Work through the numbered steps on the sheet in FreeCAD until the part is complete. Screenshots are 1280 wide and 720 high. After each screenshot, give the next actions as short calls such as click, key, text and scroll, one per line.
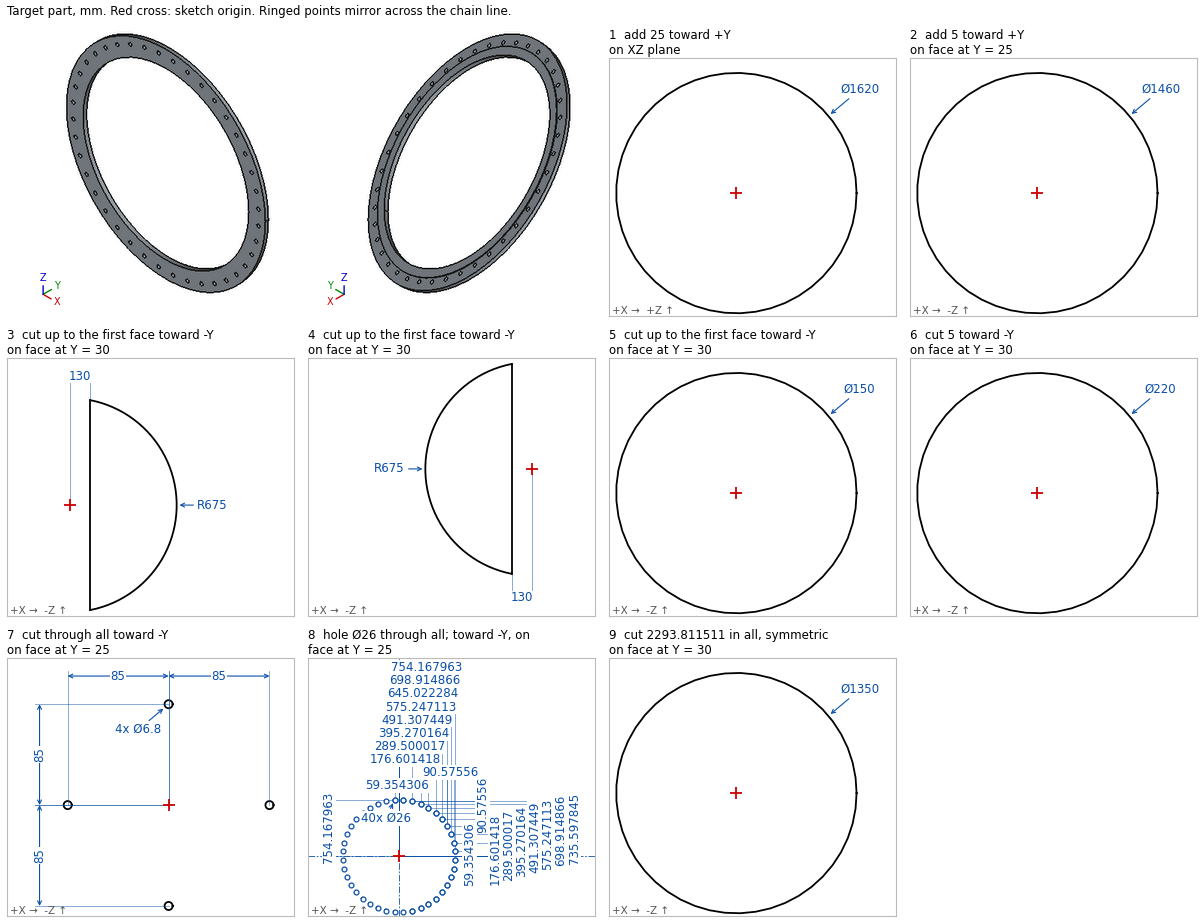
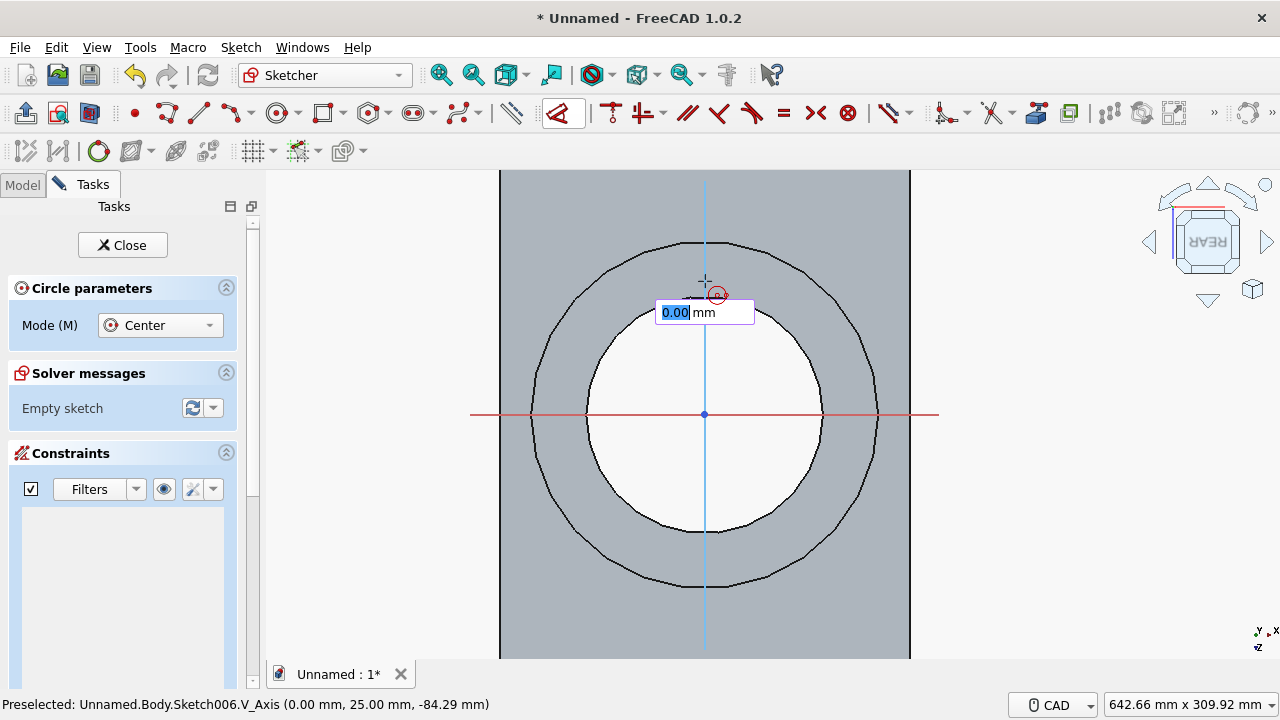
scroll(710, 279, up, 6)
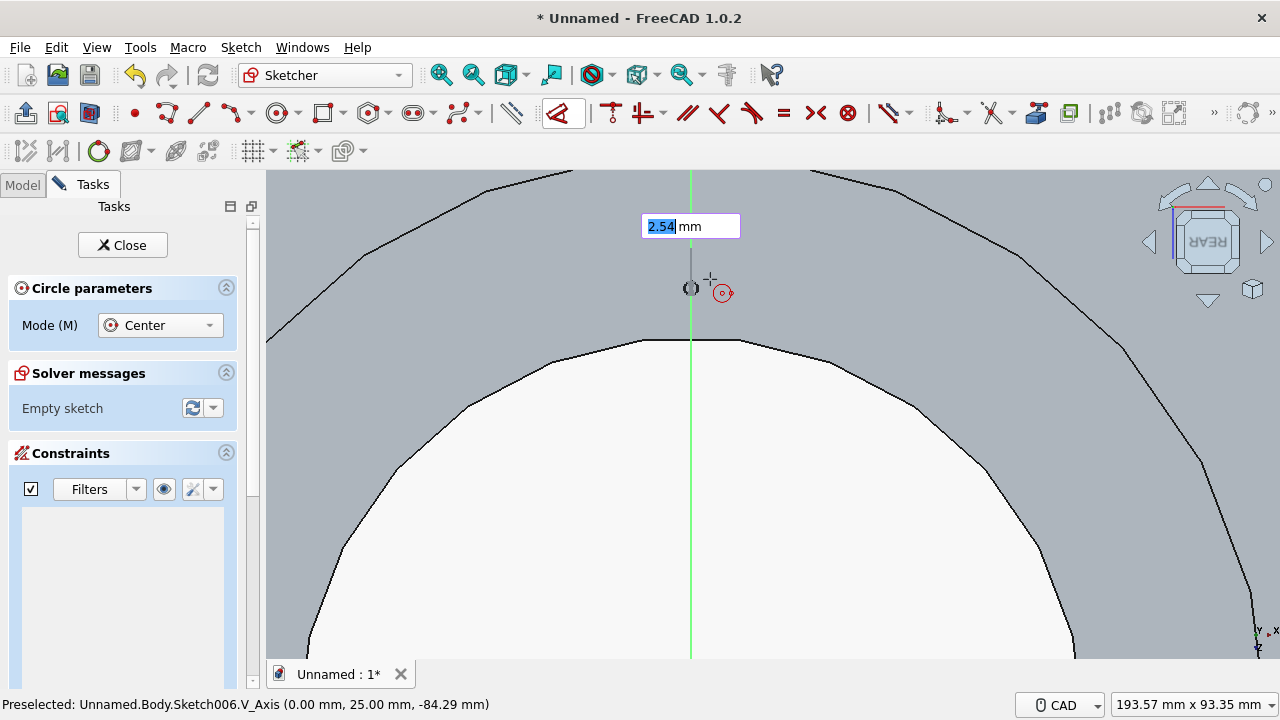
click(708, 279)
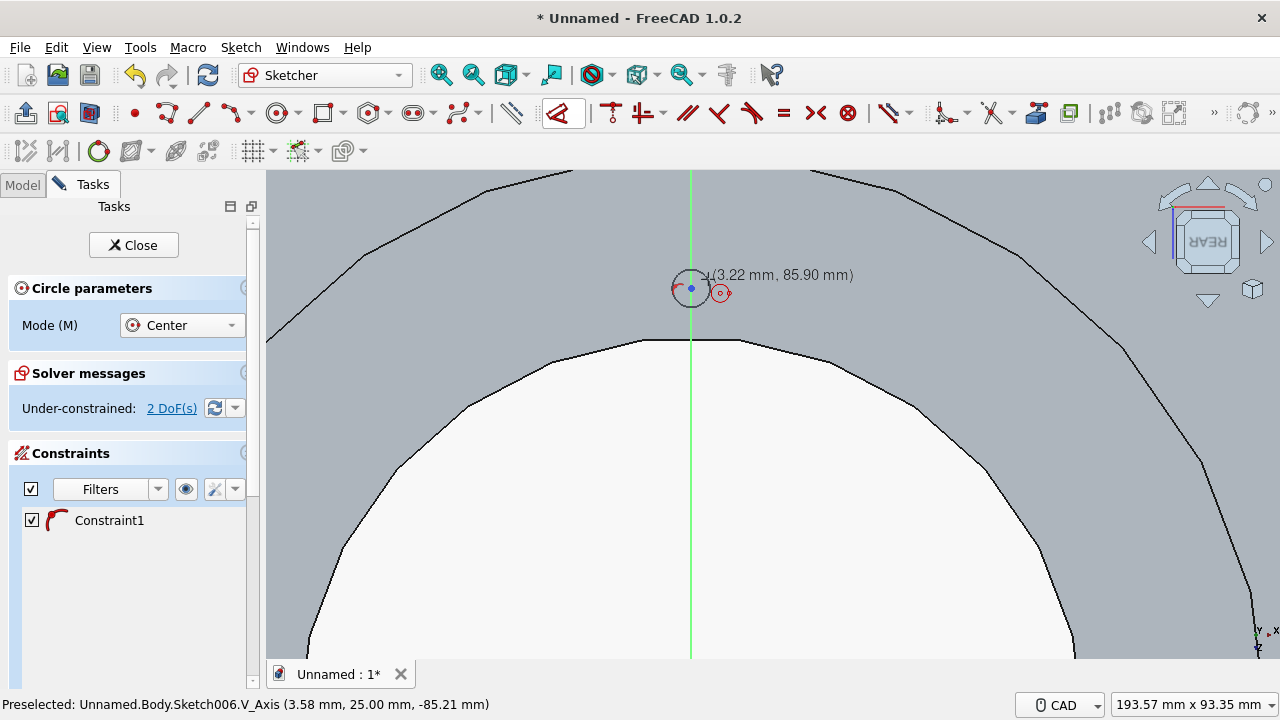
scroll(710, 279, down, 6)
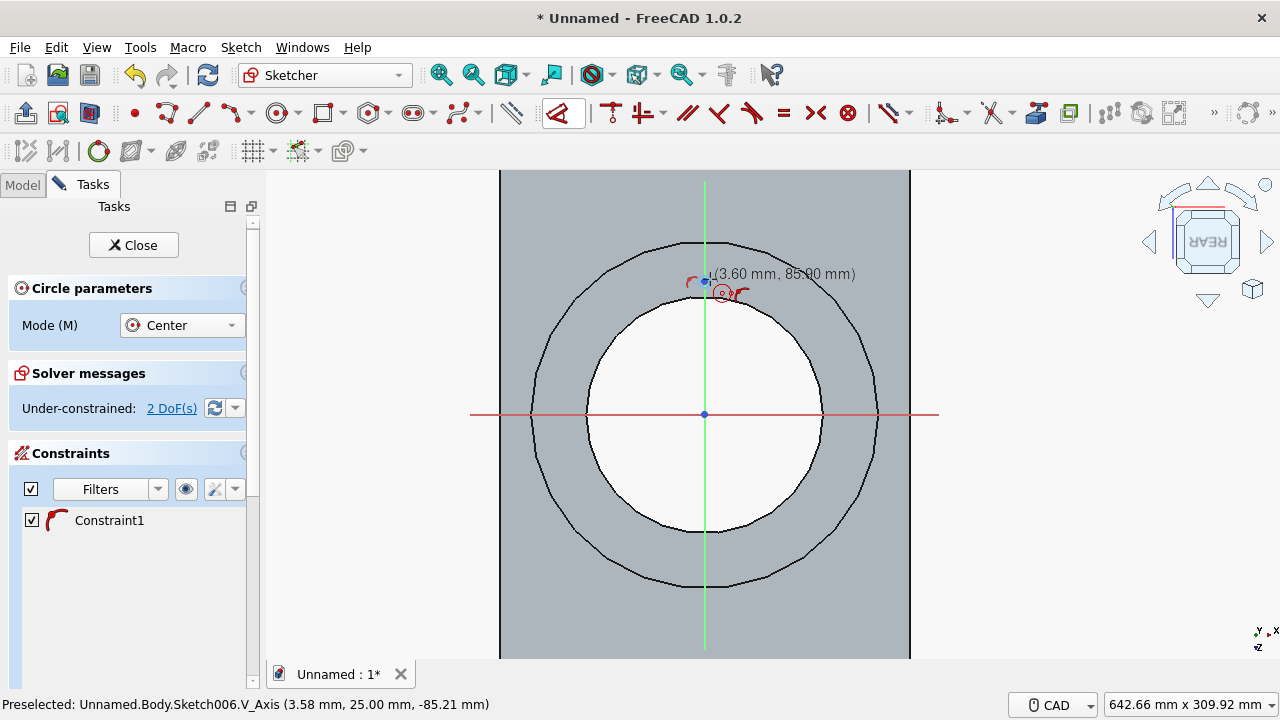
scroll(839, 415, up, 8)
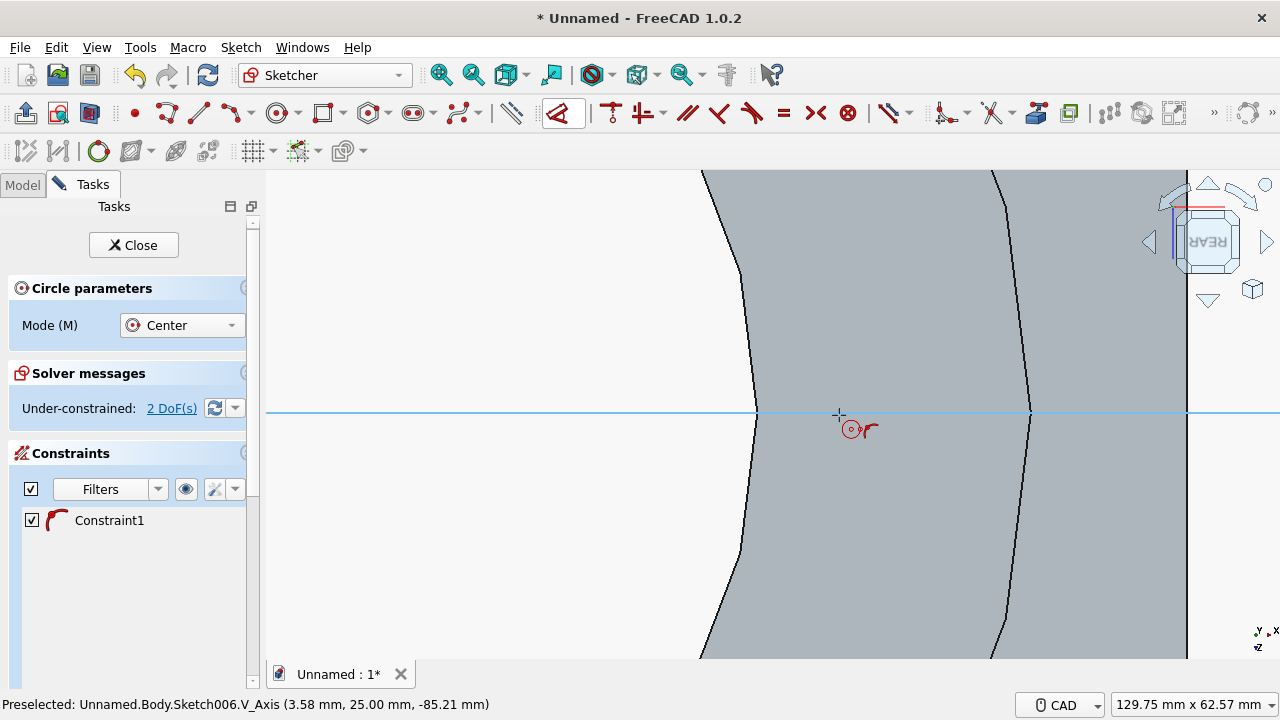
scroll(839, 415, down, 8)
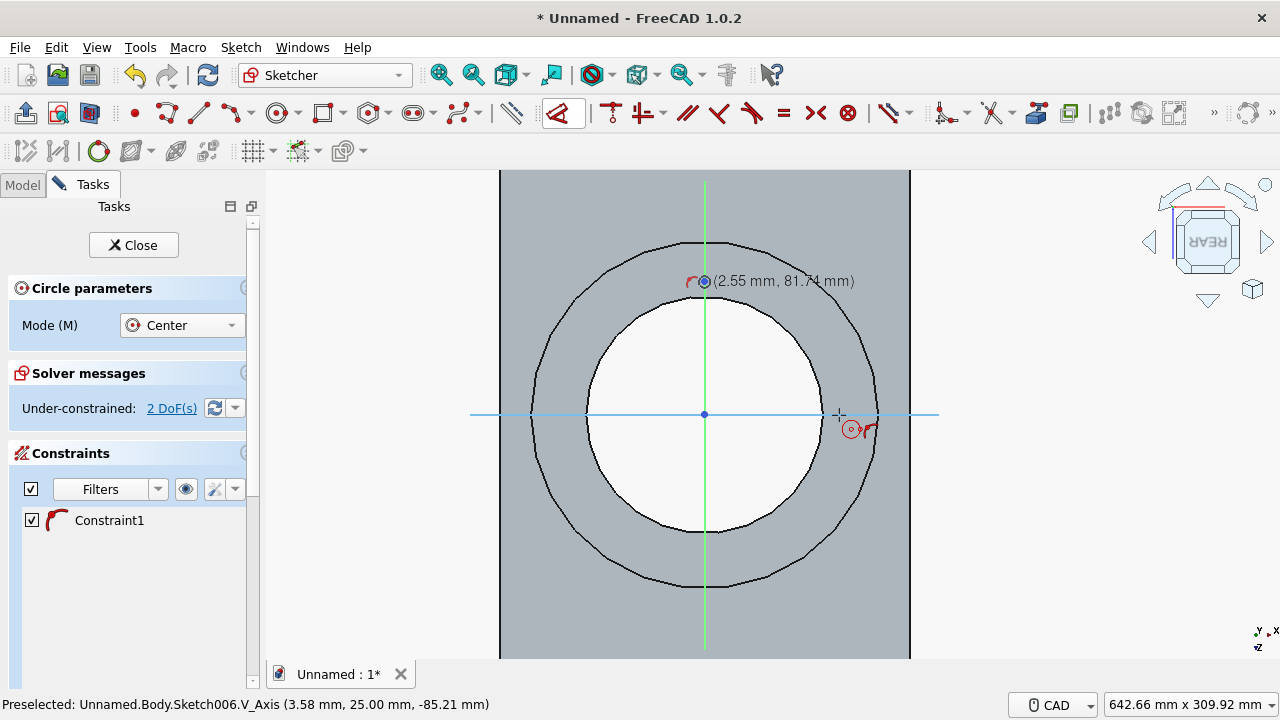
click(839, 415)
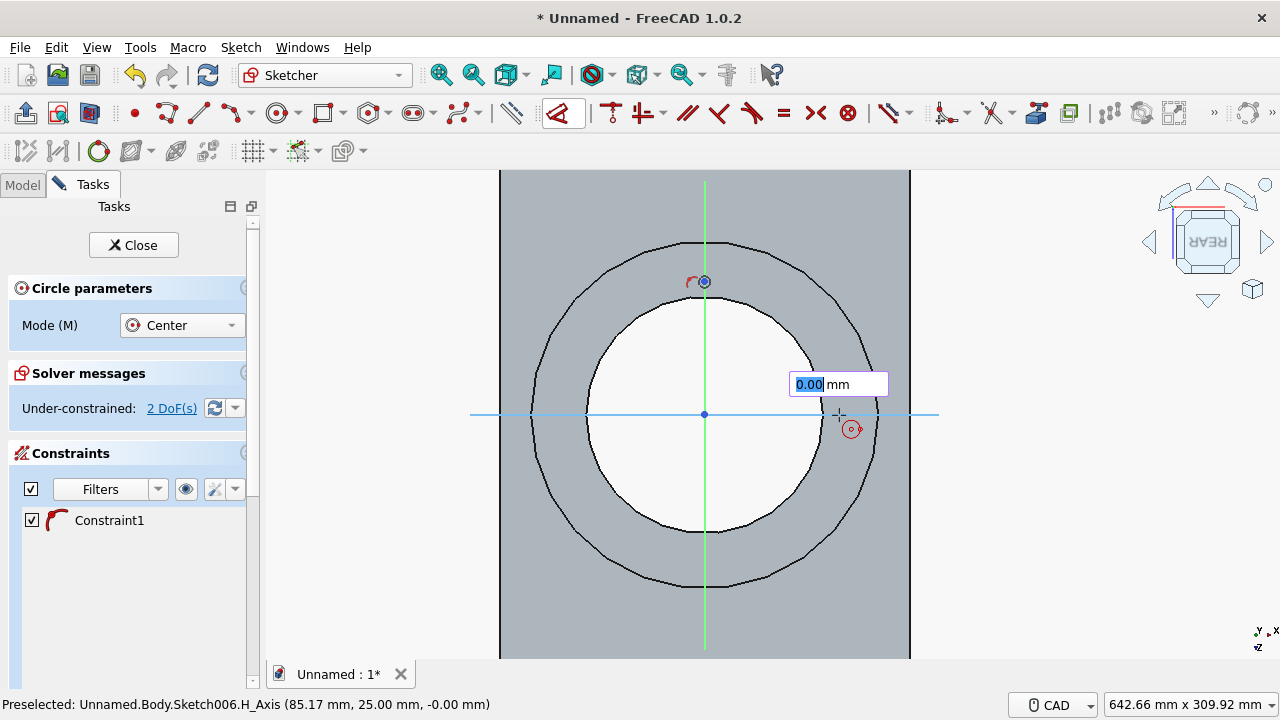
scroll(837, 420, up, 6)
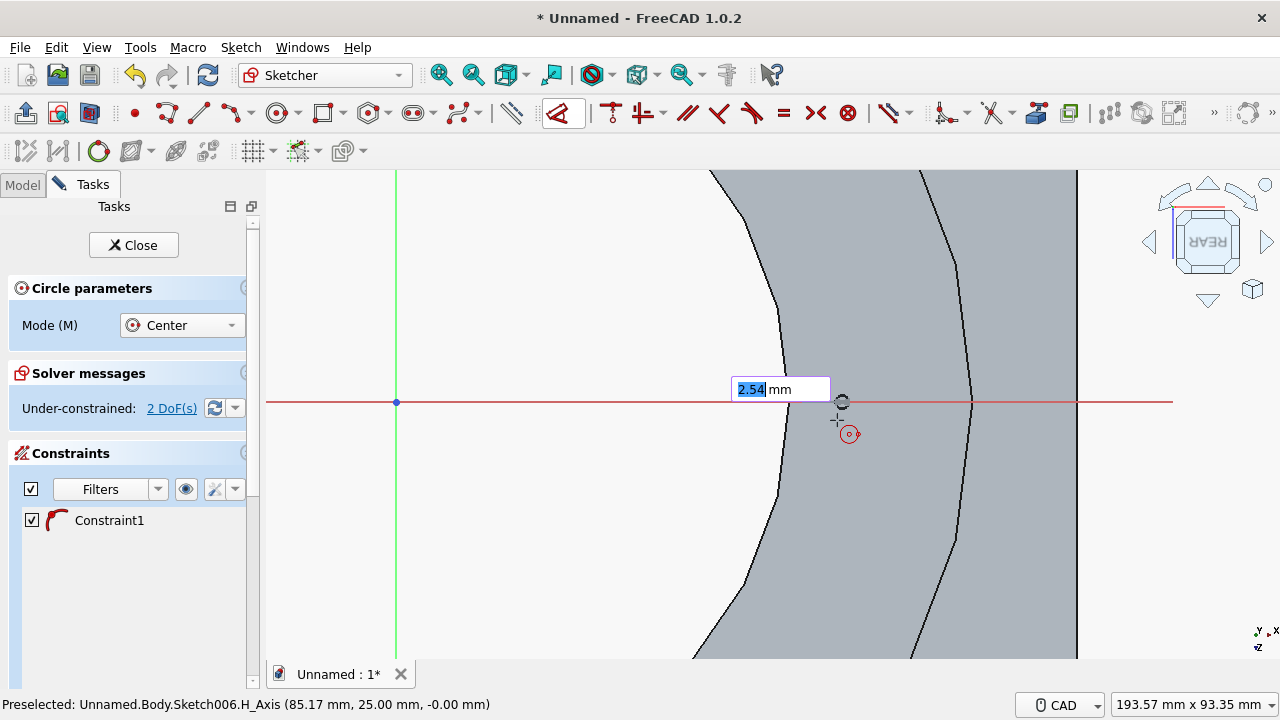
click(835, 419)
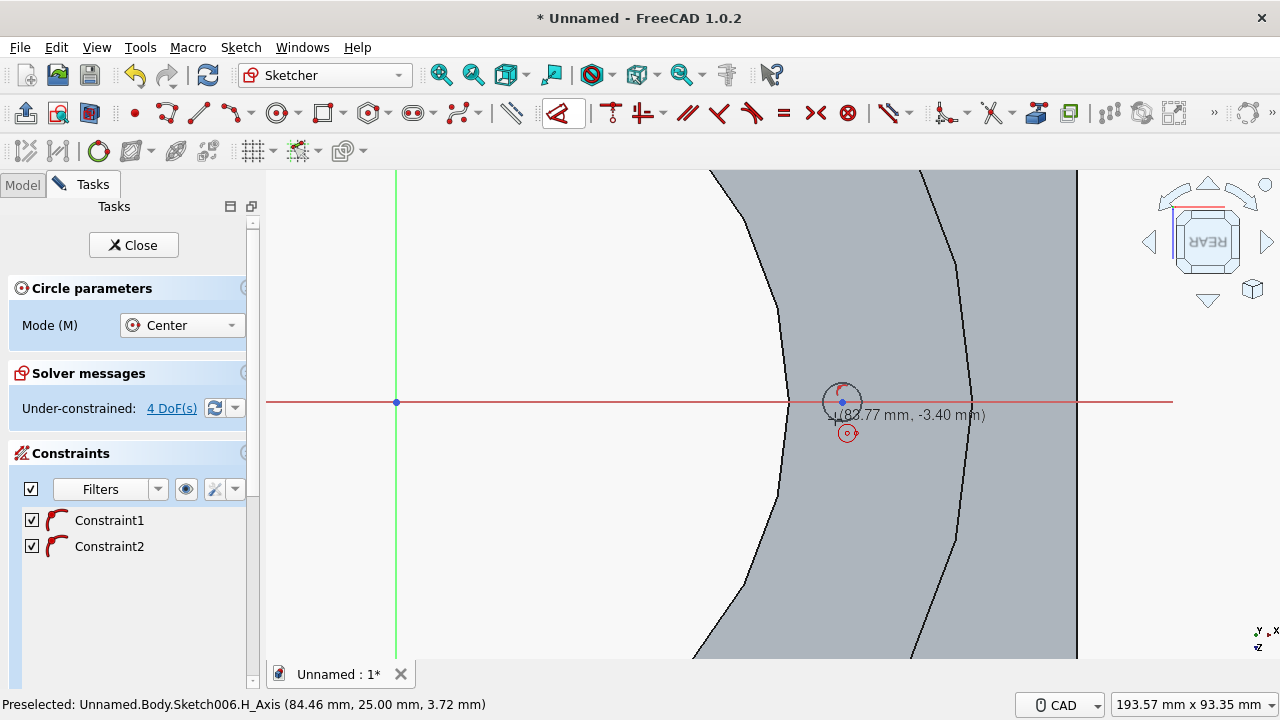
scroll(837, 420, down, 6)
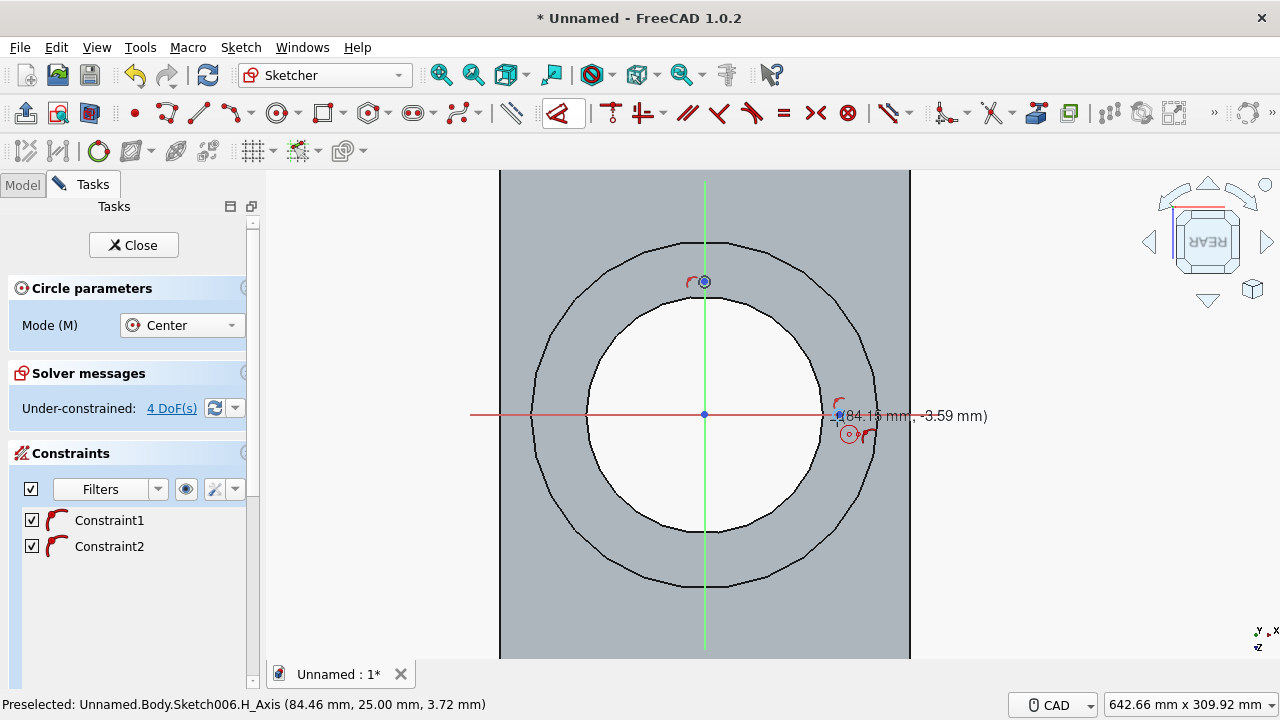
scroll(705, 549, up, 8)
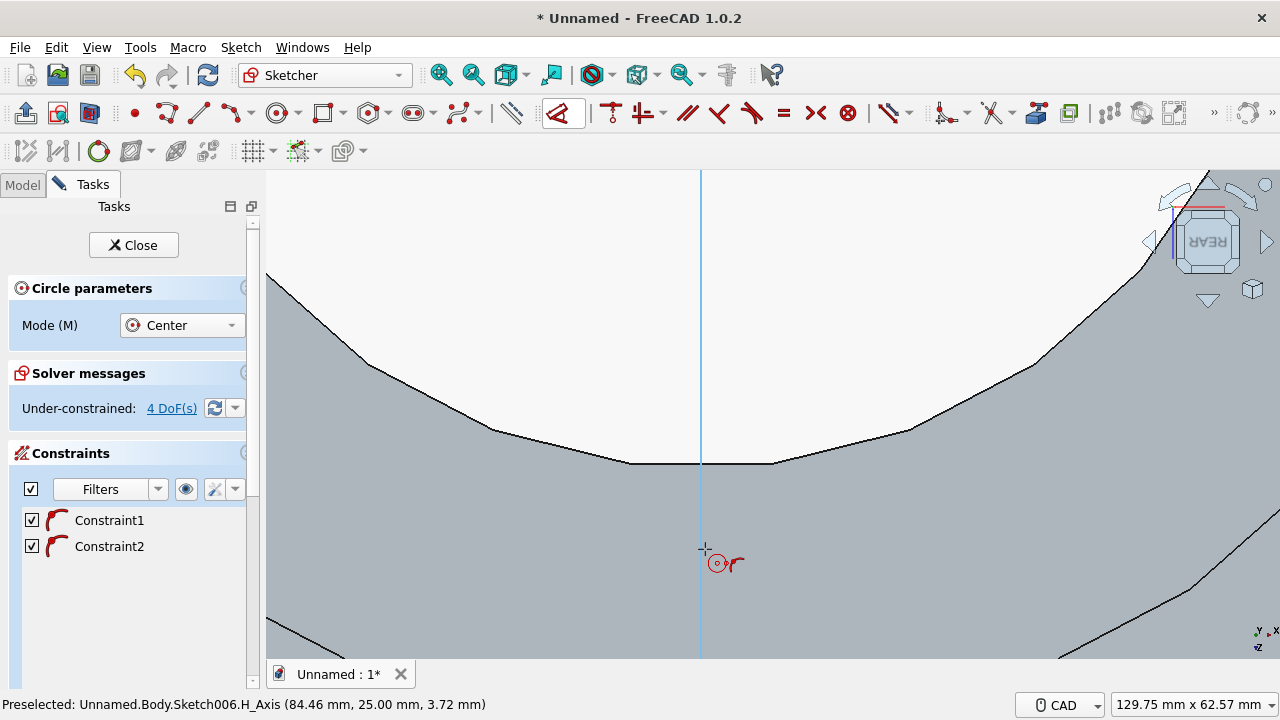
scroll(705, 549, down, 8)